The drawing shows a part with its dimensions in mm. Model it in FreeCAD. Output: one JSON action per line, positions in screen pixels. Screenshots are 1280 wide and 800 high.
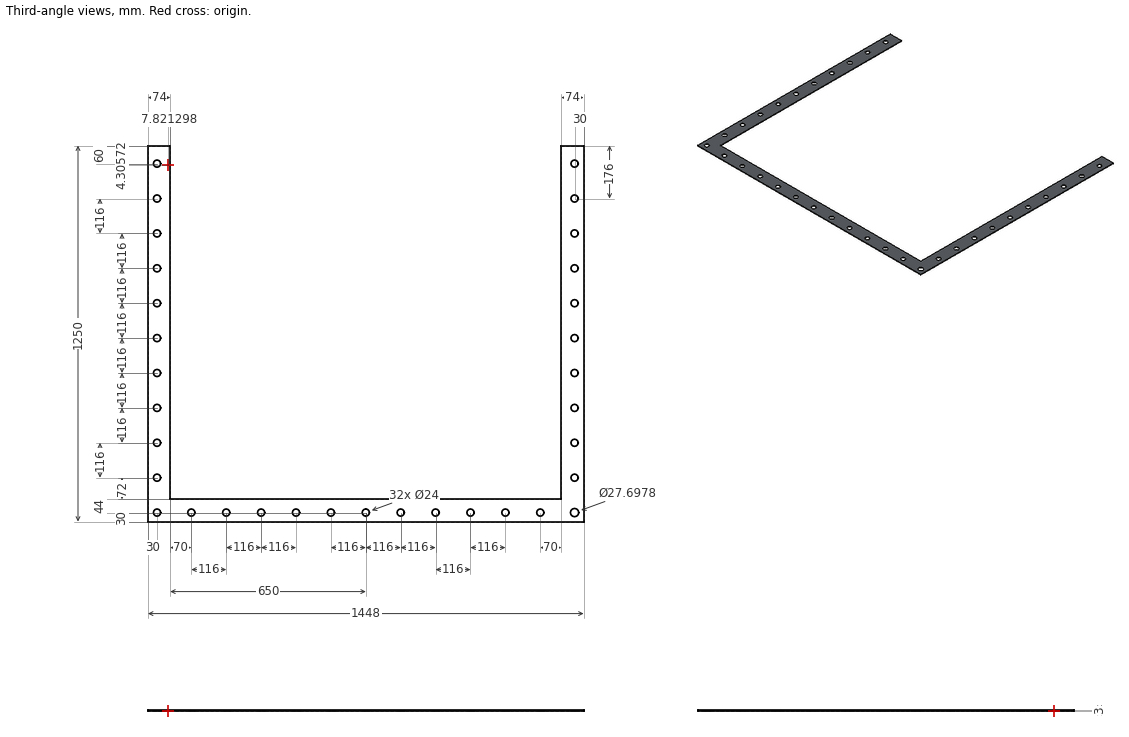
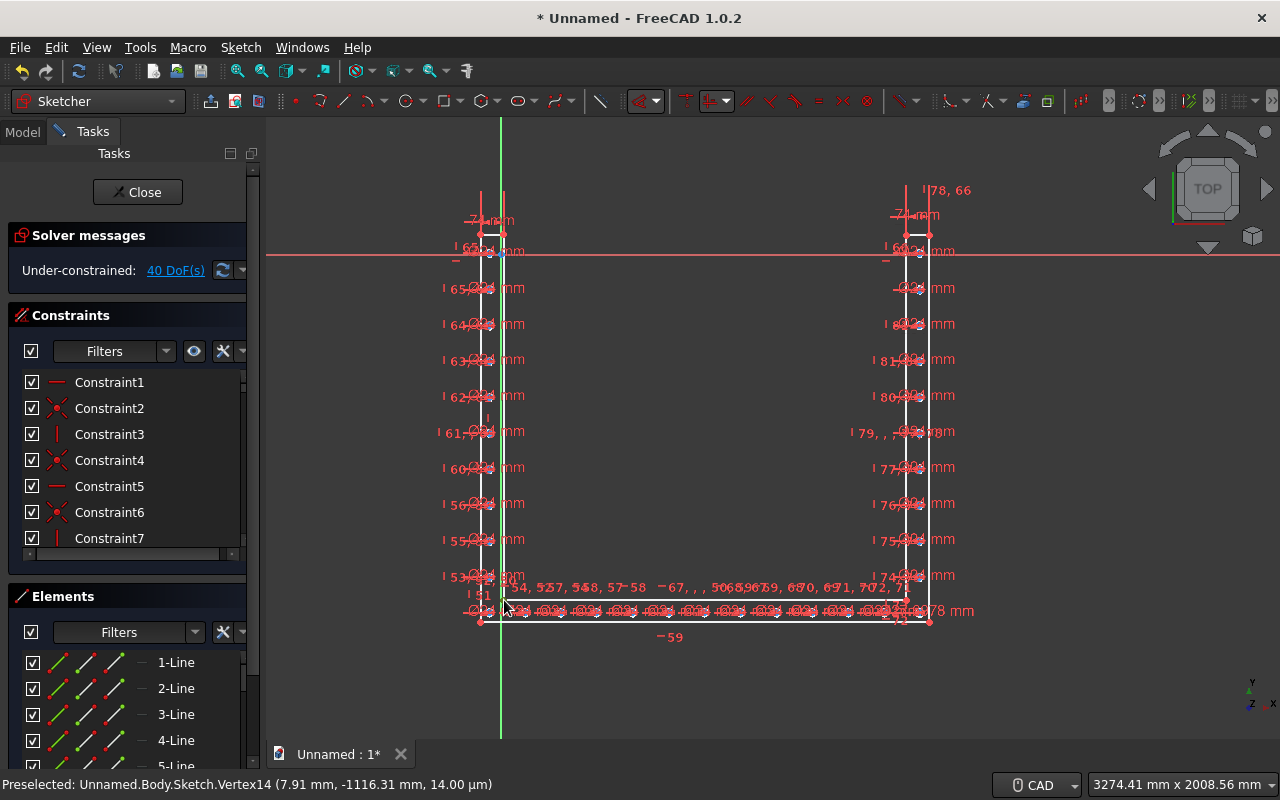
{"action": "scroll", "coordinate": [705, 613], "scroll_direction": "up", "scroll_amount": 6}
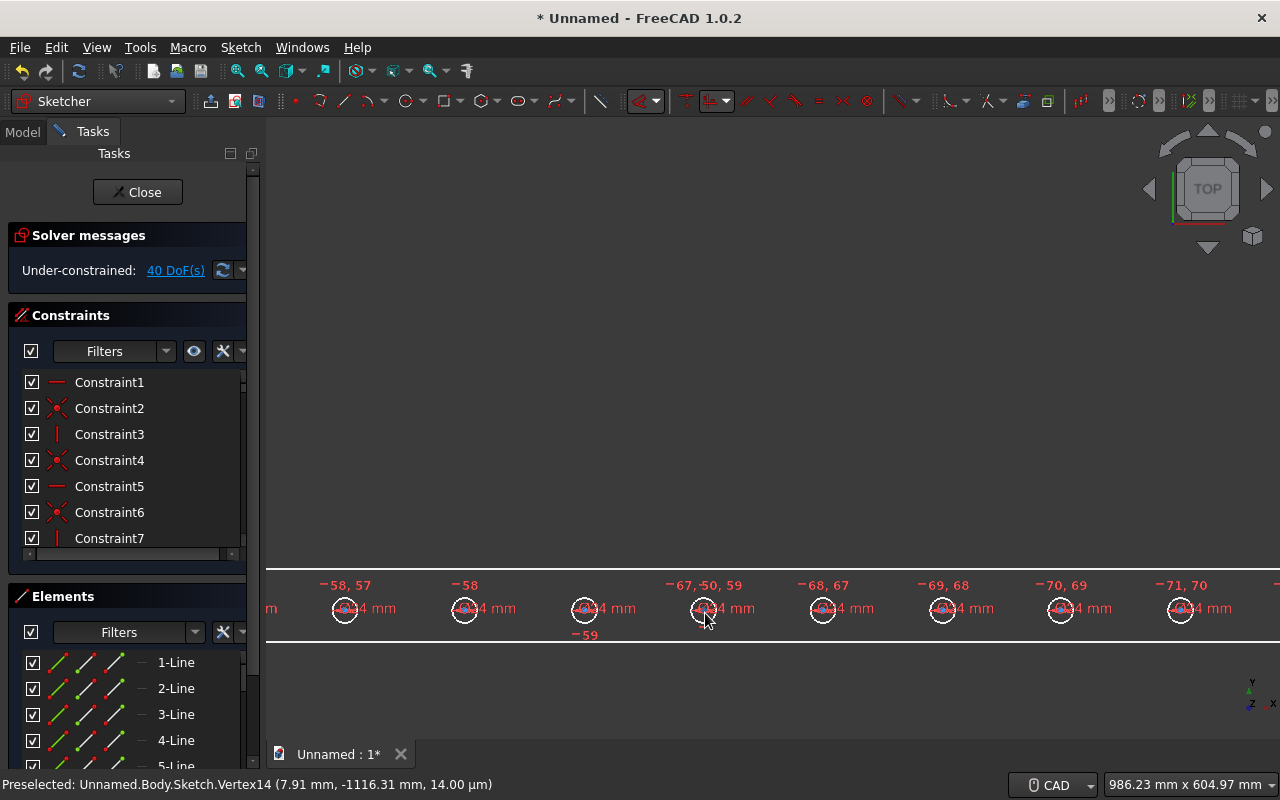
{"action": "left_click", "coordinate": [704, 611]}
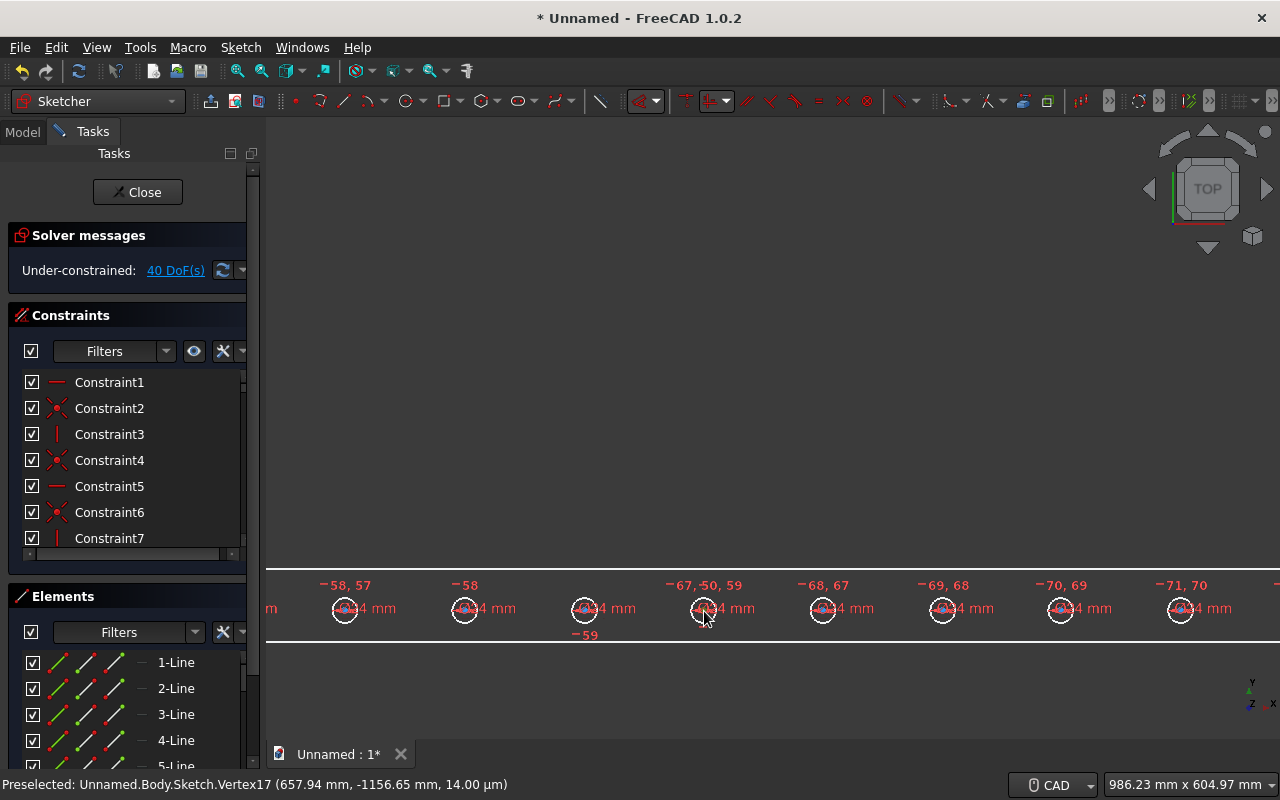
{"action": "left_click", "coordinate": [658, 102]}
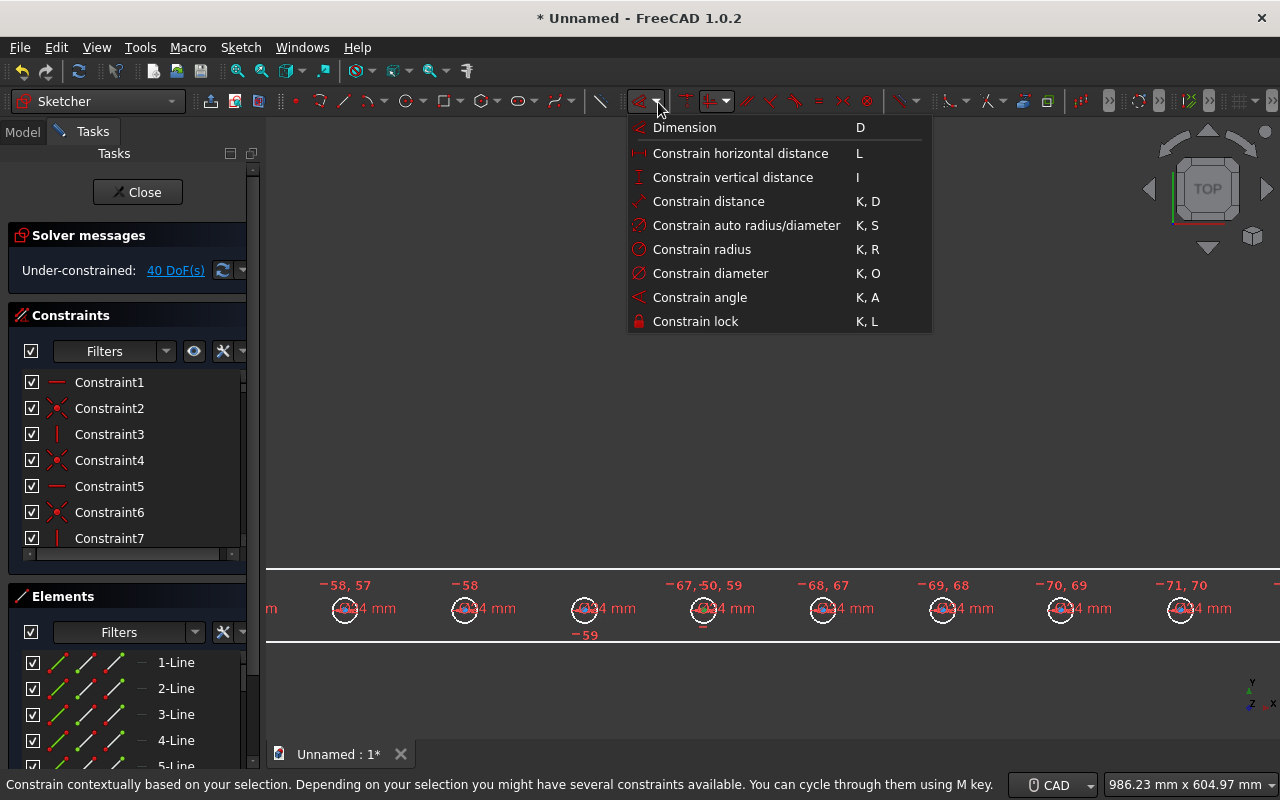
{"action": "left_click", "coordinate": [780, 177]}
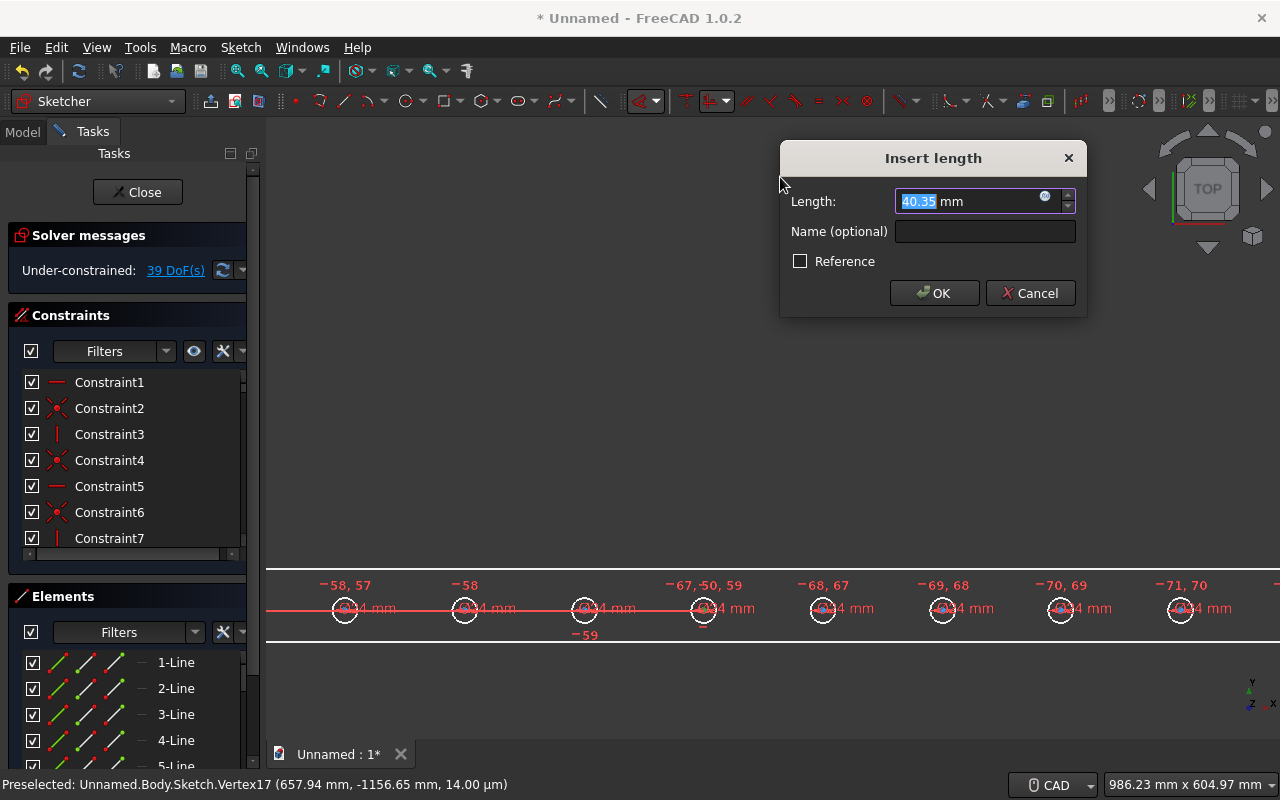
{"action": "type", "text": "44"}
{"action": "key", "text": "Return"}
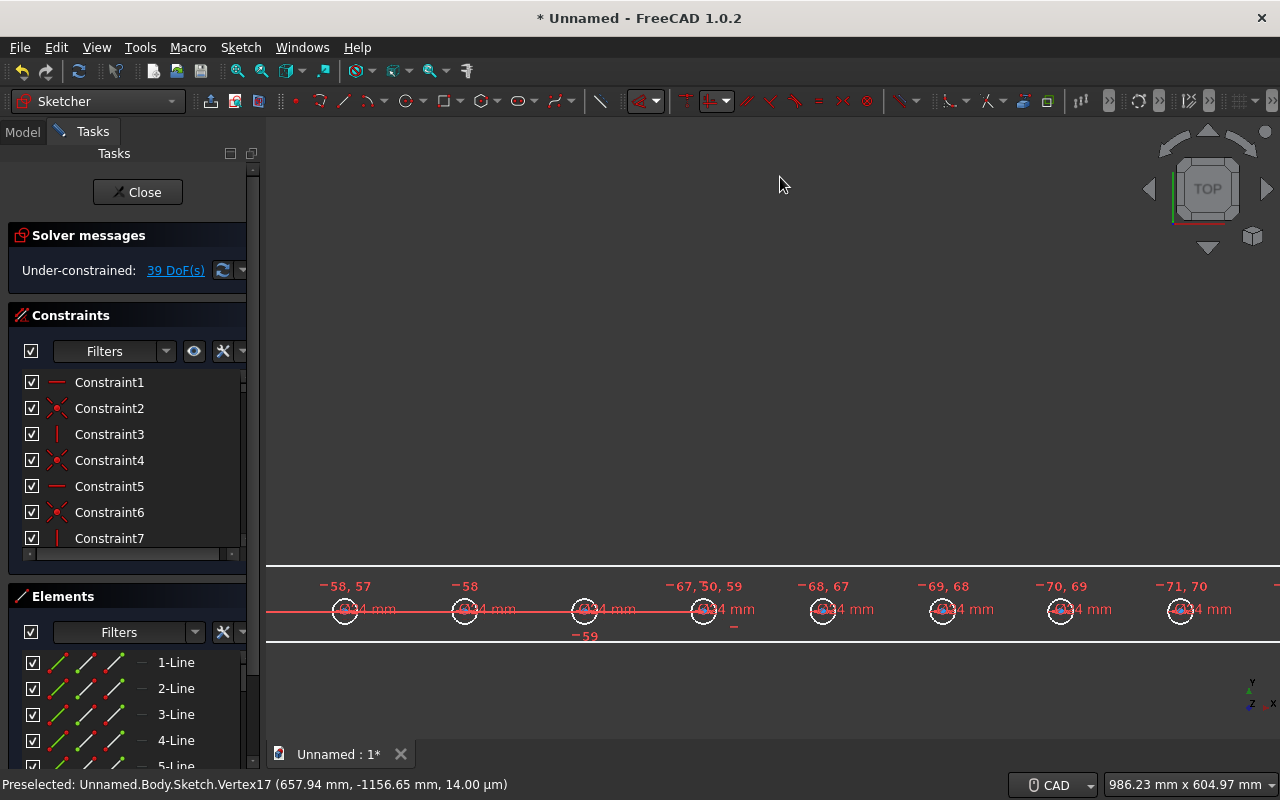
{"action": "scroll", "coordinate": [705, 613], "scroll_direction": "down", "scroll_amount": 6}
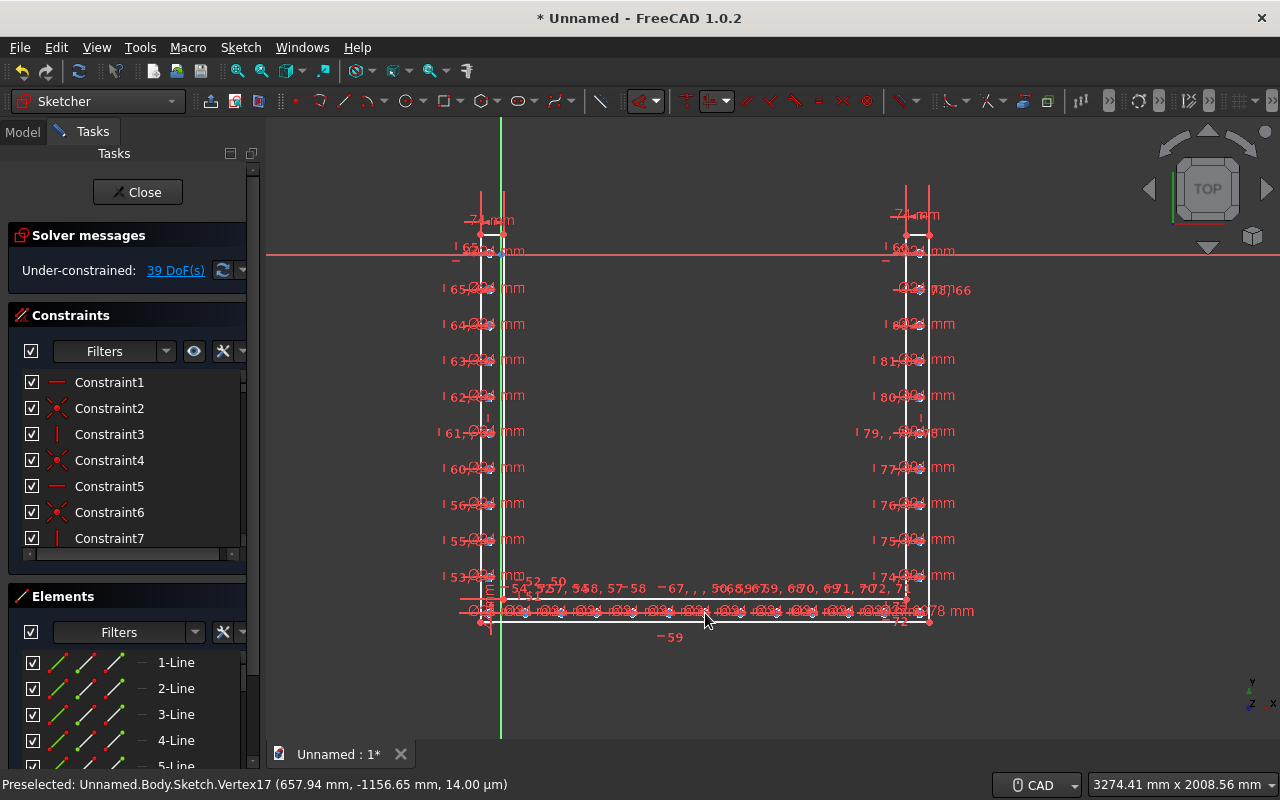
{"action": "scroll", "coordinate": [481, 622], "scroll_direction": "up", "scroll_amount": 8}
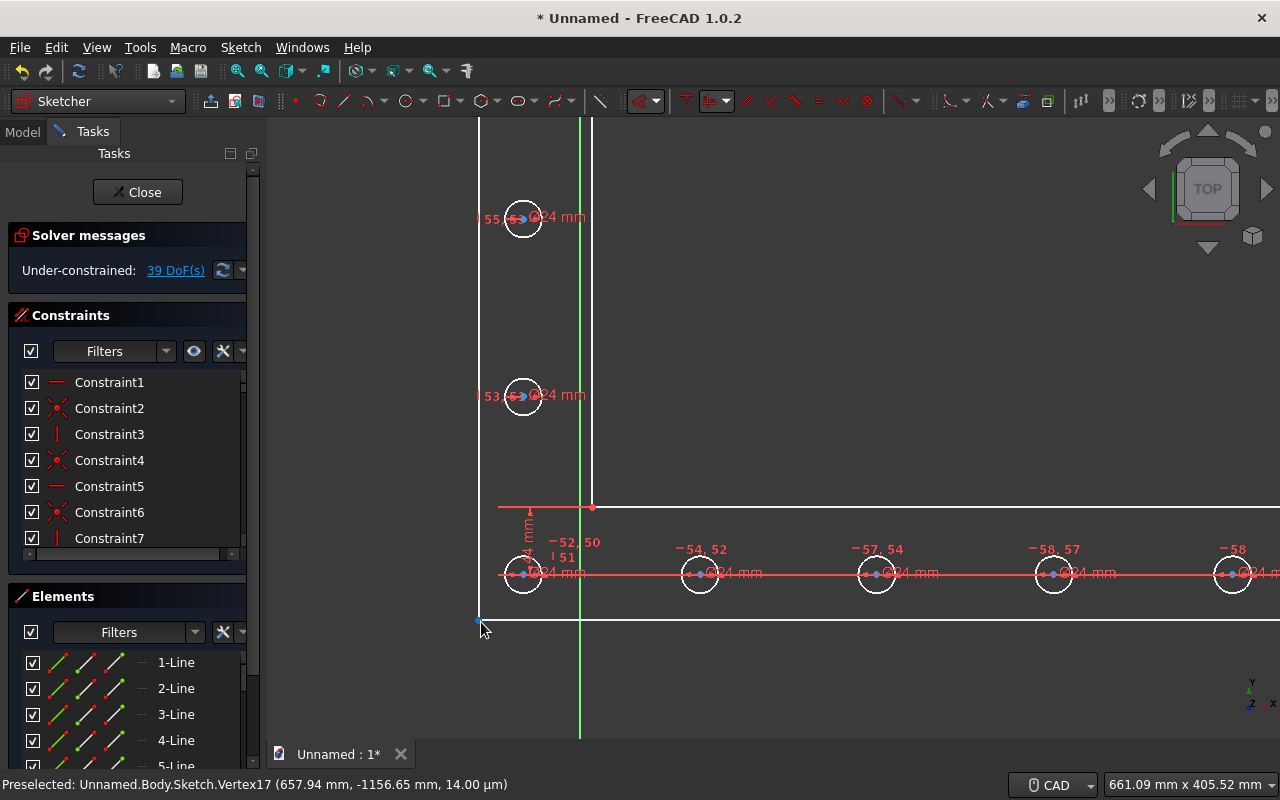
{"action": "left_click", "coordinate": [479, 620]}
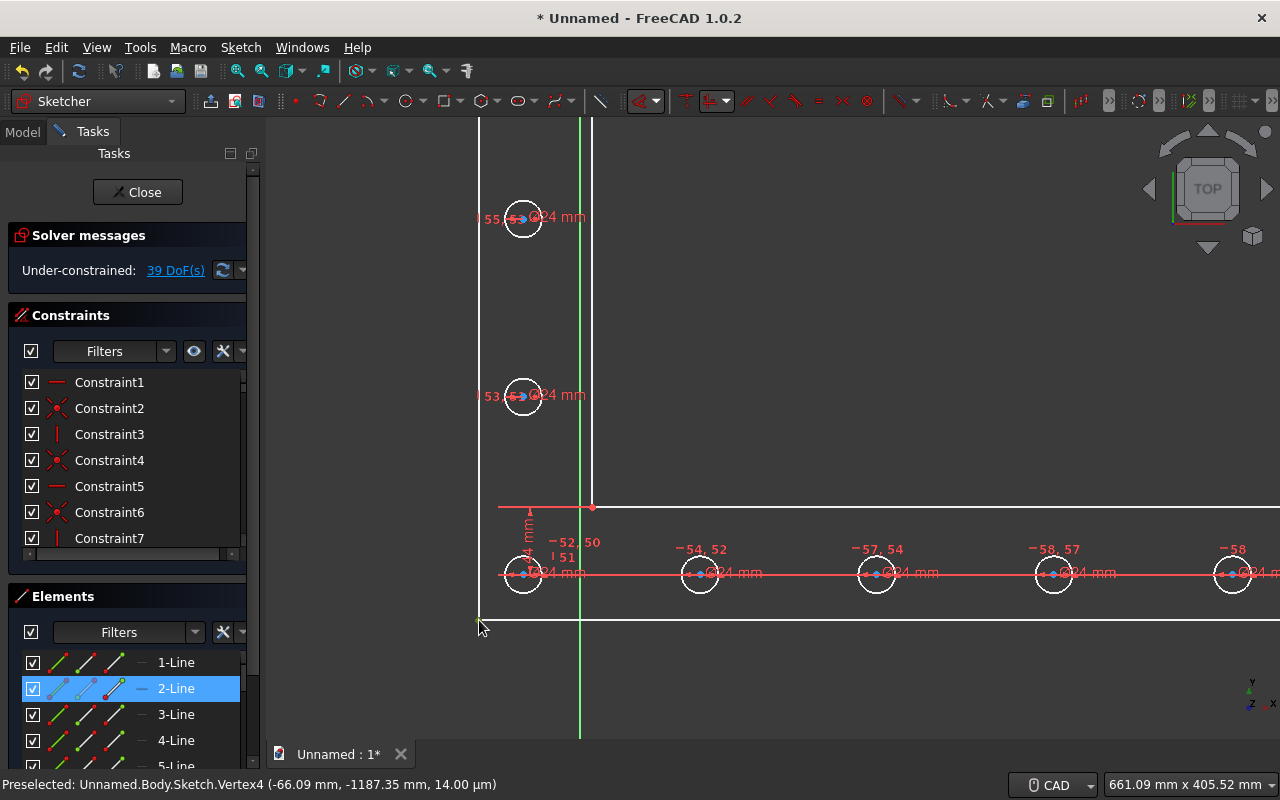
{"action": "scroll", "coordinate": [481, 622], "scroll_direction": "down", "scroll_amount": 8}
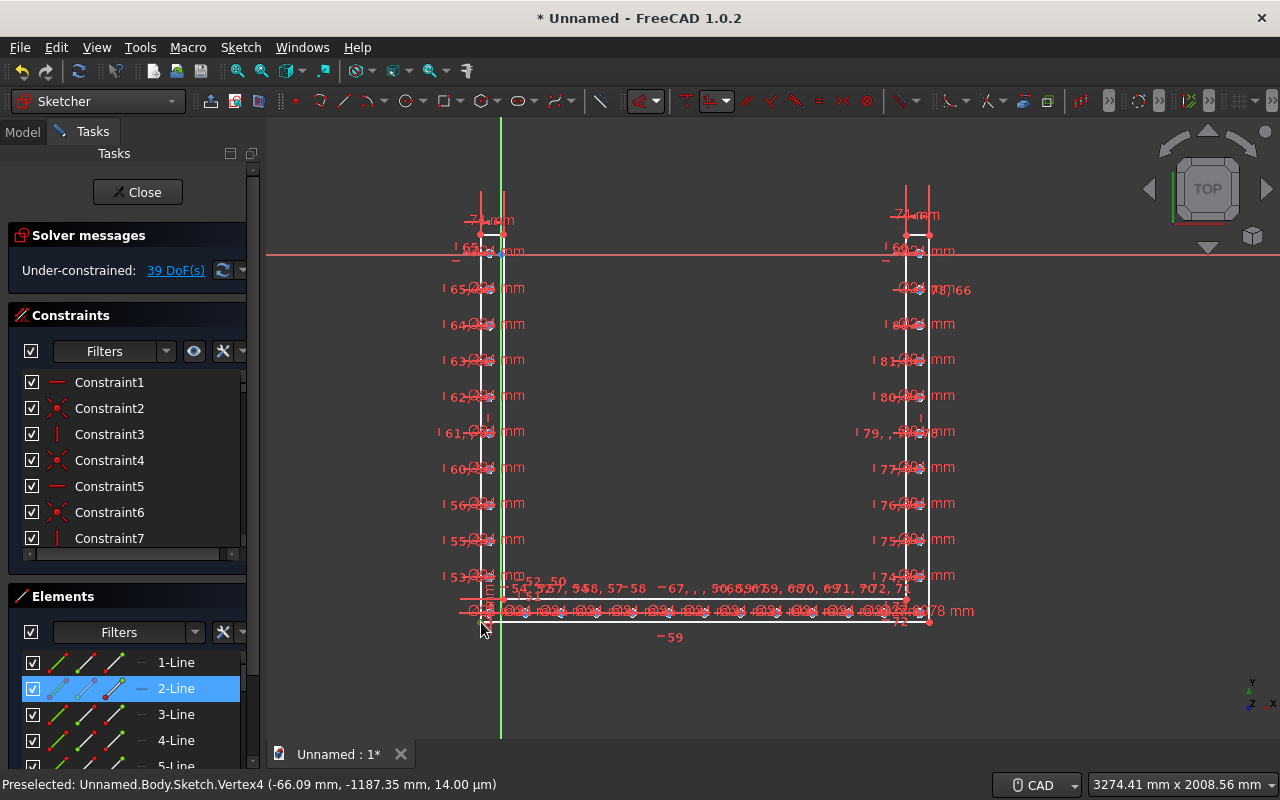
{"action": "scroll", "coordinate": [705, 613], "scroll_direction": "up", "scroll_amount": 8}